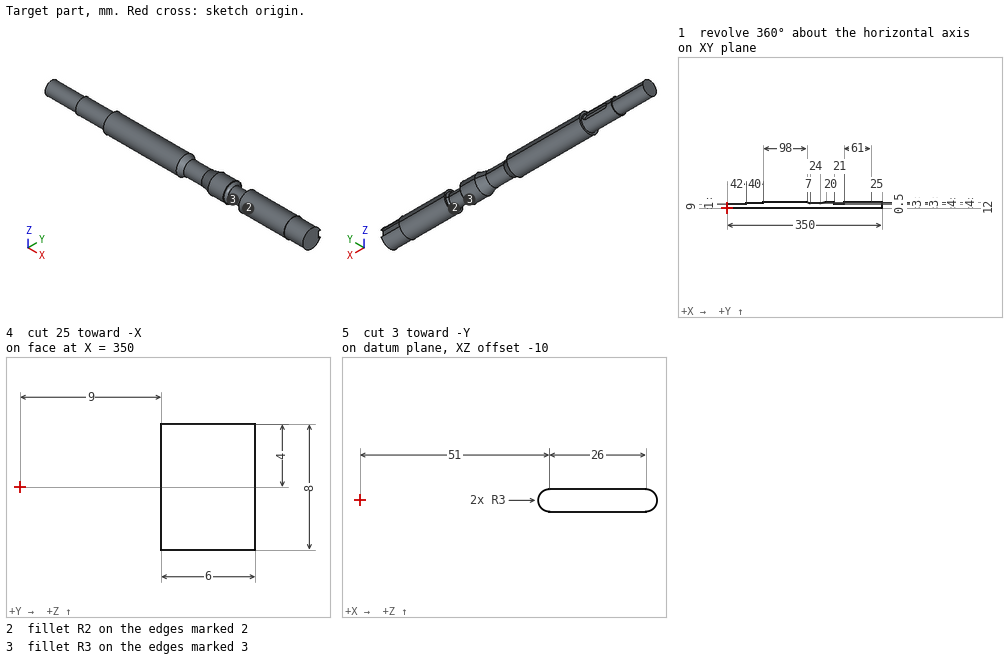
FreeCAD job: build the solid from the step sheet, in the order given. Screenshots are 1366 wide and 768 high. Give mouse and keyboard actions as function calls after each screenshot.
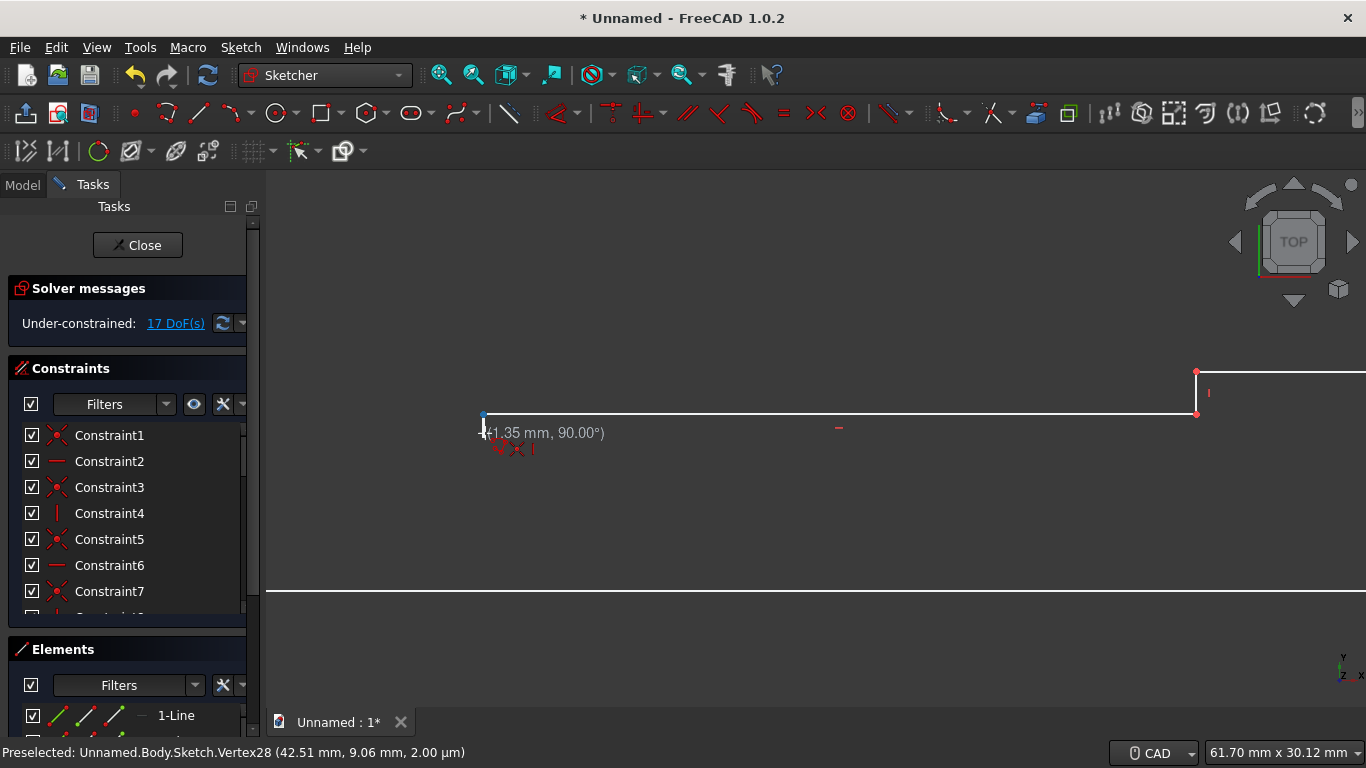
click(483, 430)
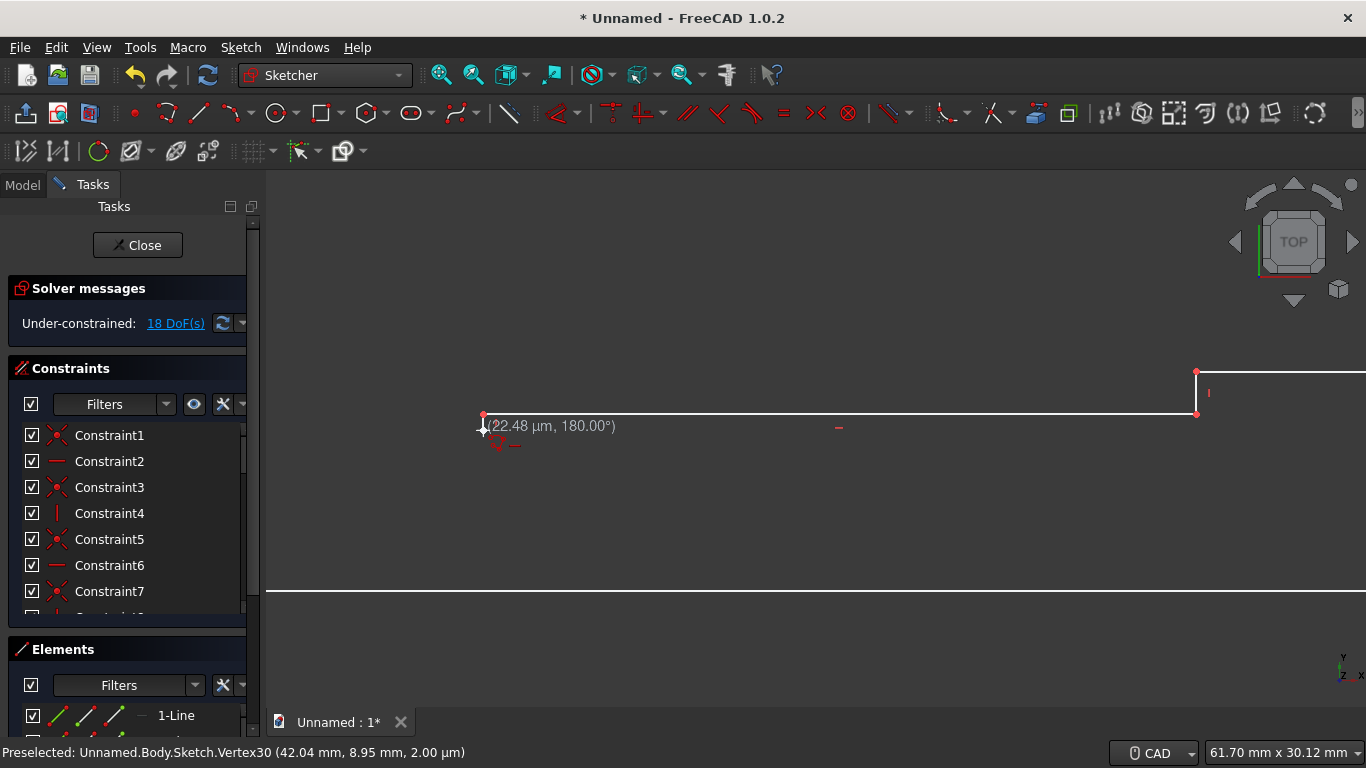
scroll(485, 433, down, 11)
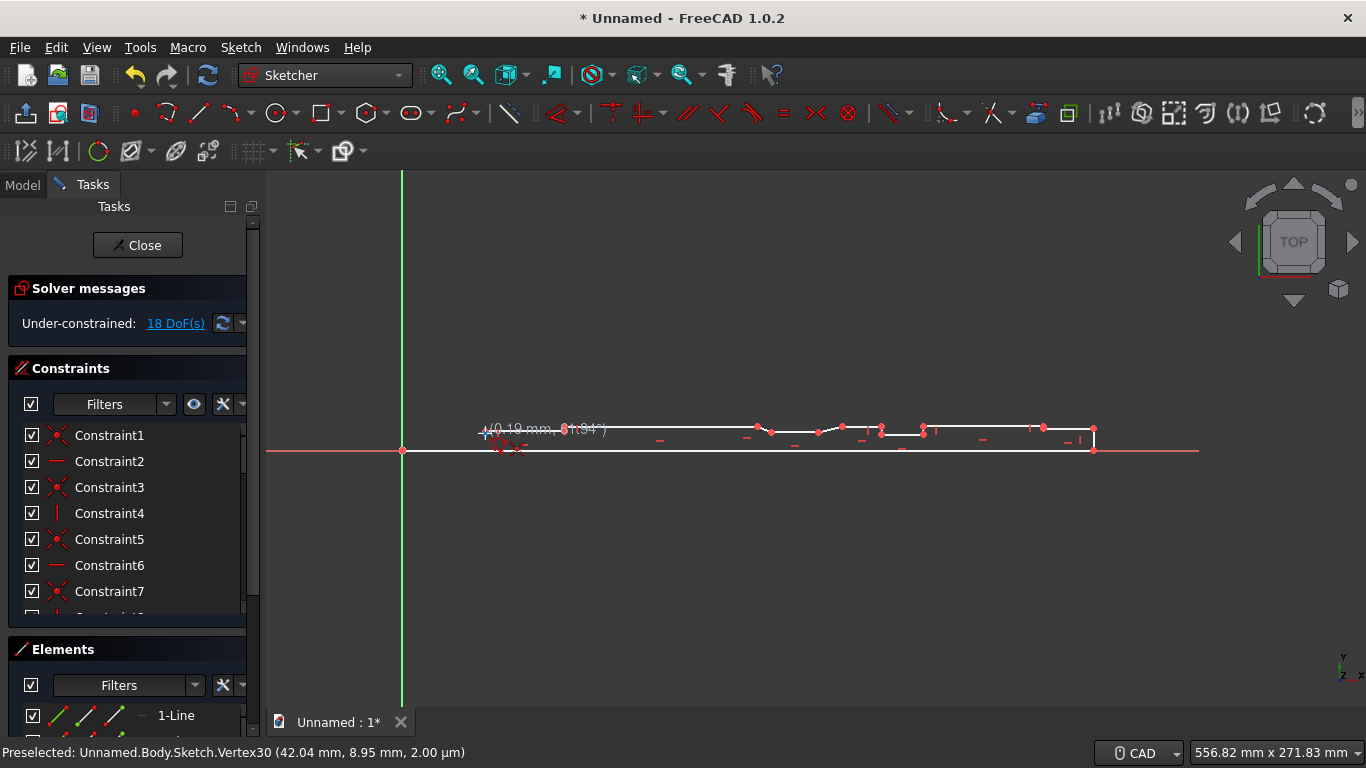
click(411, 433)
click(402, 451)
key(Escape)
key(Escape)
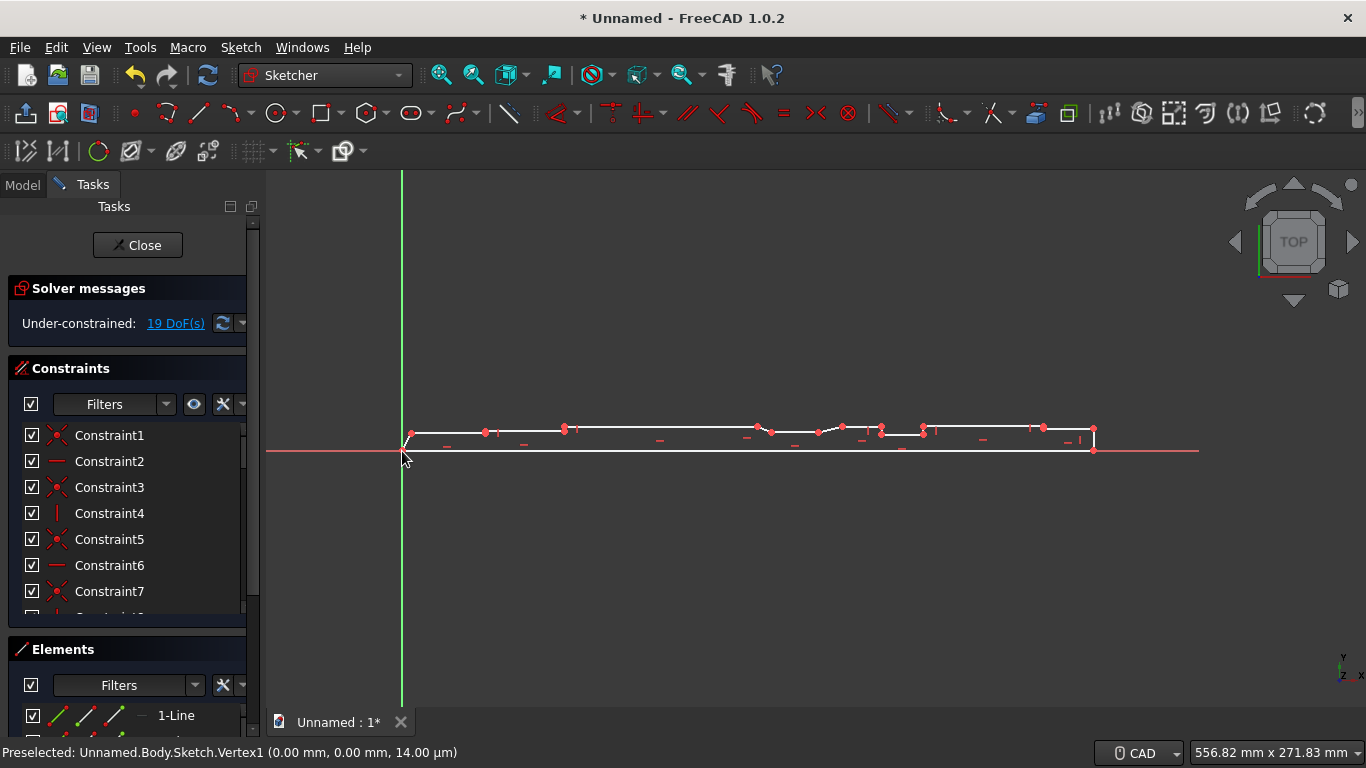
scroll(406, 444, up, 4)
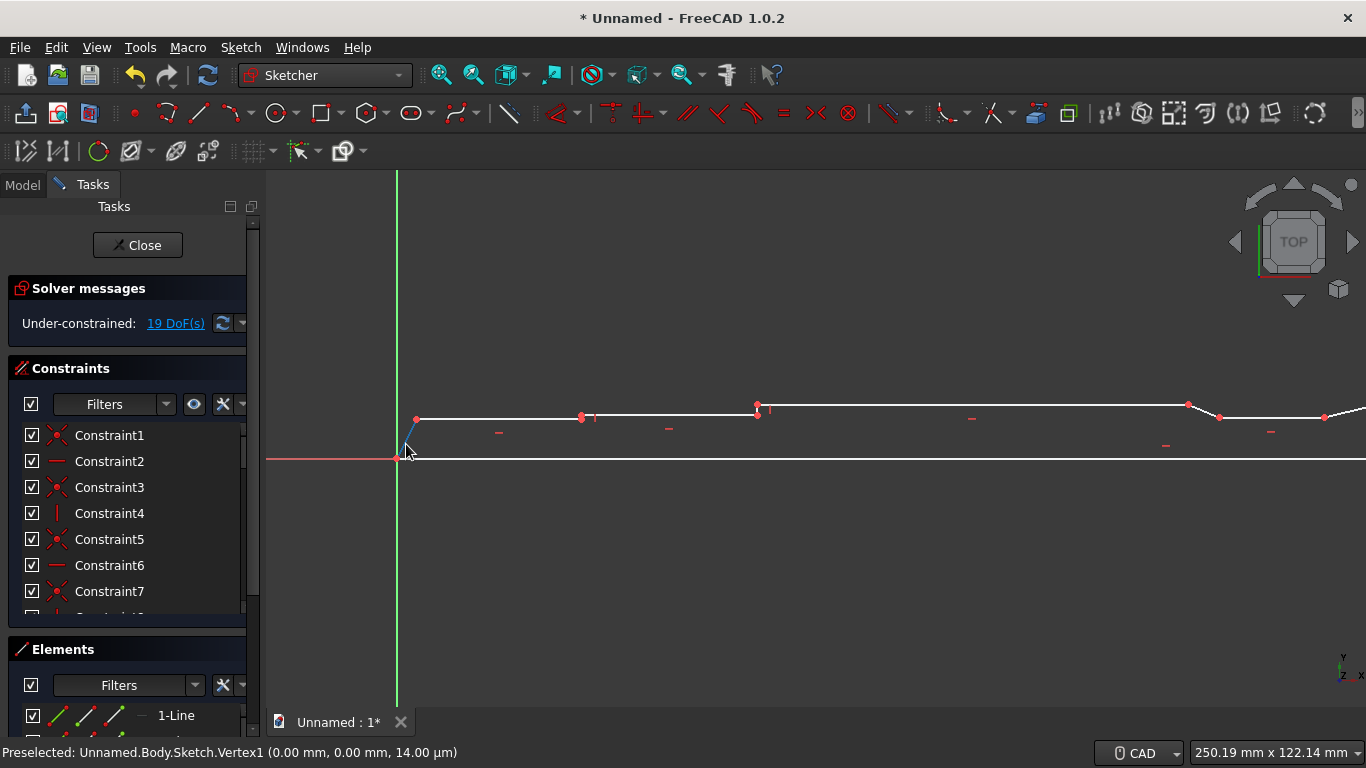
click(405, 443)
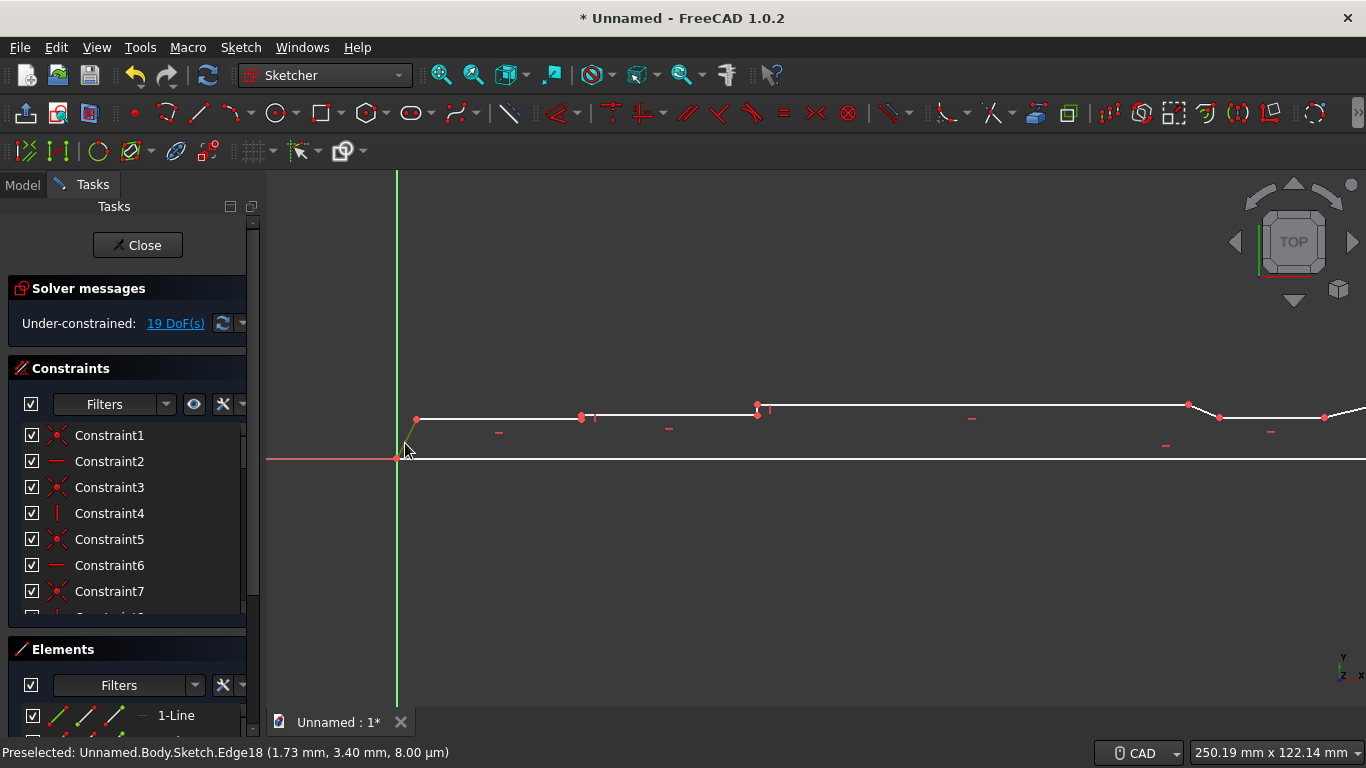
key(v)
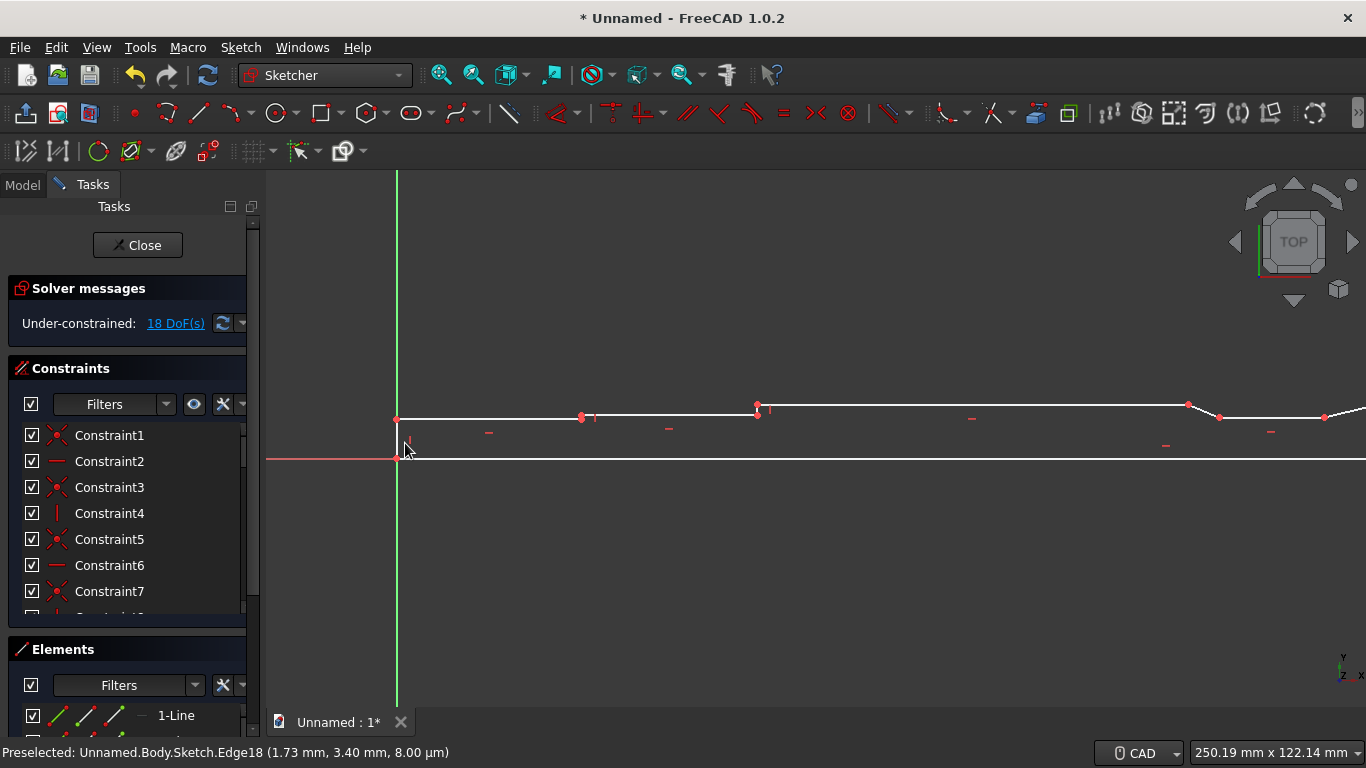
click(556, 114)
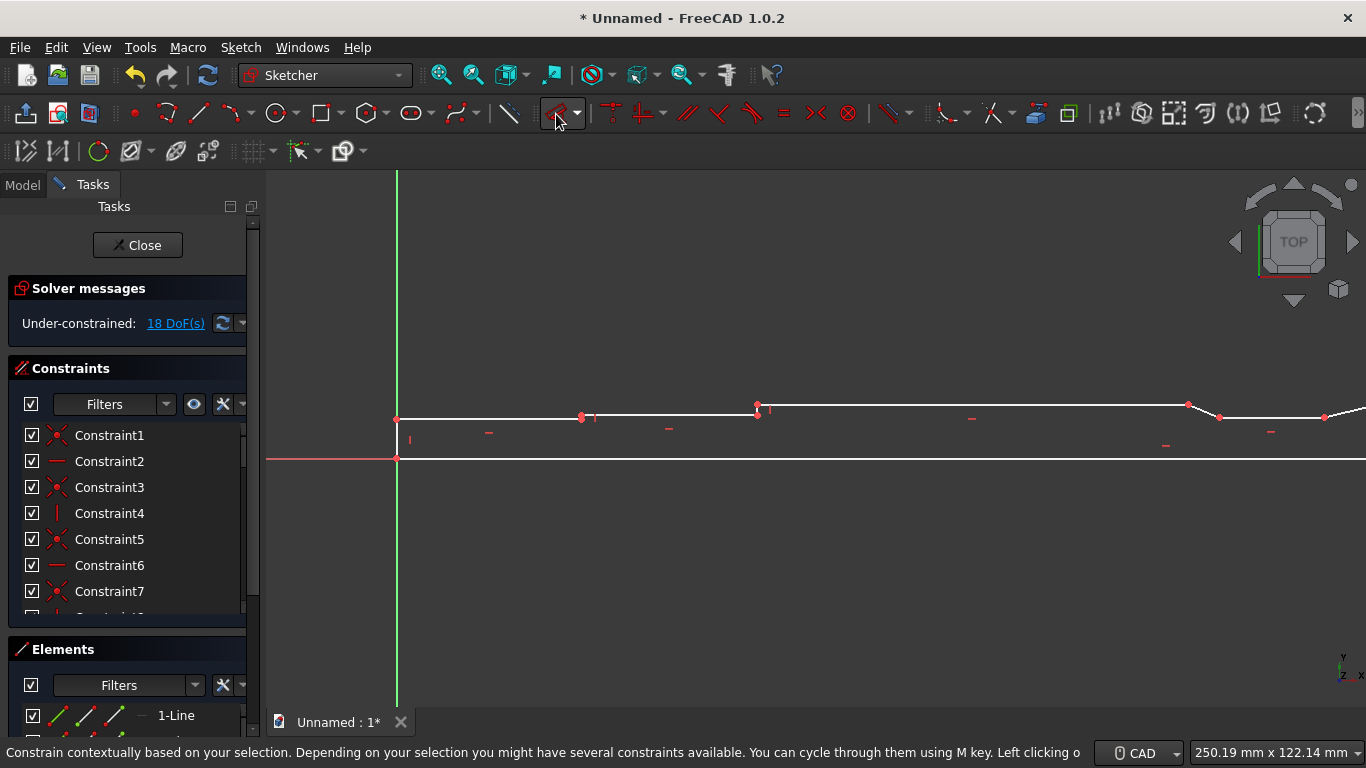
scroll(406, 444, down, 4)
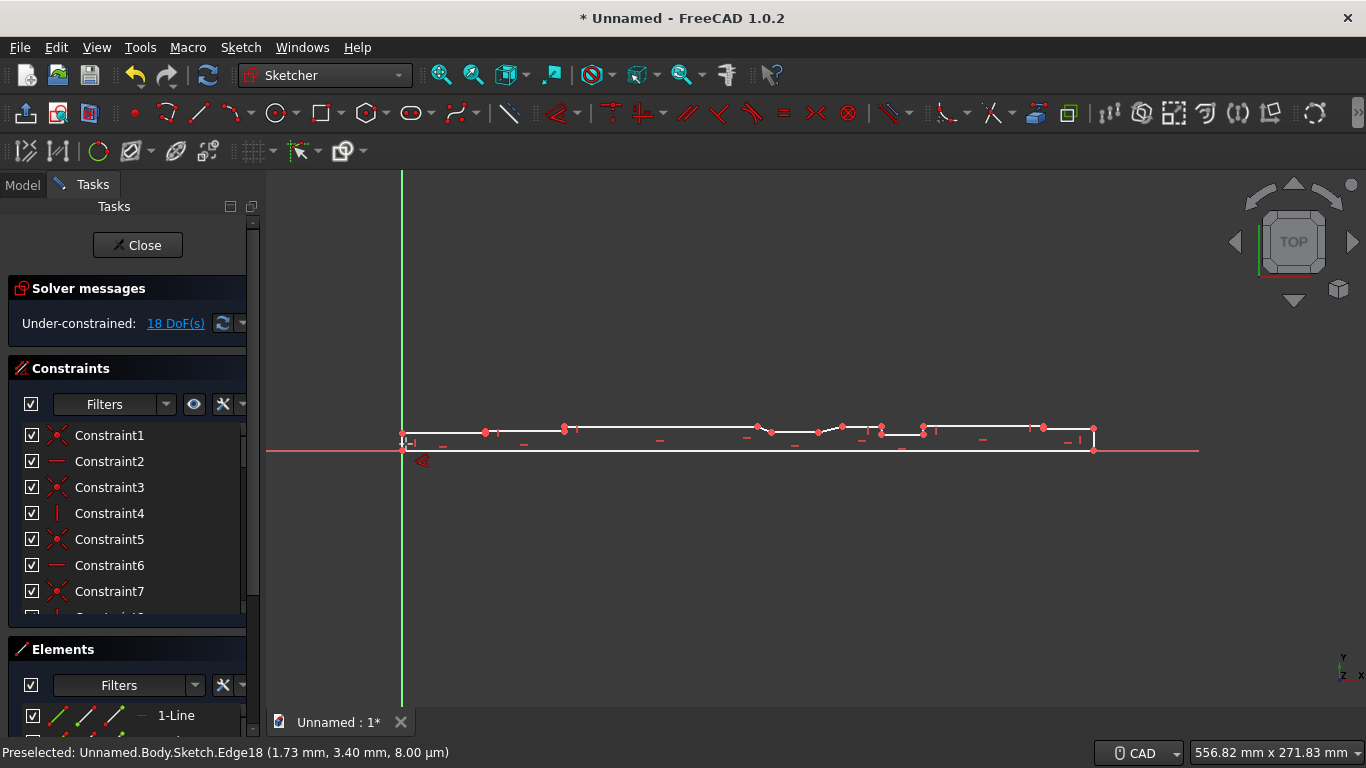
scroll(923, 430, up, 9)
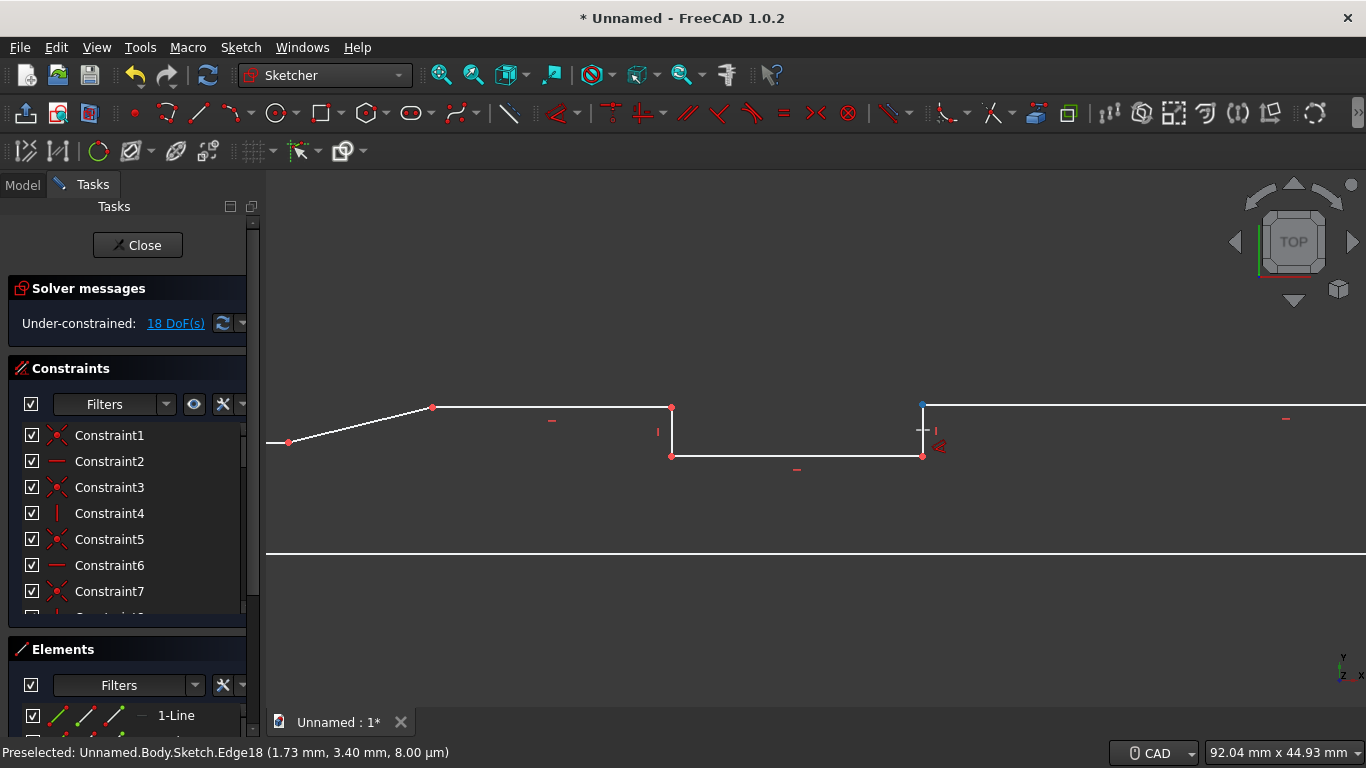
click(923, 430)
click(957, 430)